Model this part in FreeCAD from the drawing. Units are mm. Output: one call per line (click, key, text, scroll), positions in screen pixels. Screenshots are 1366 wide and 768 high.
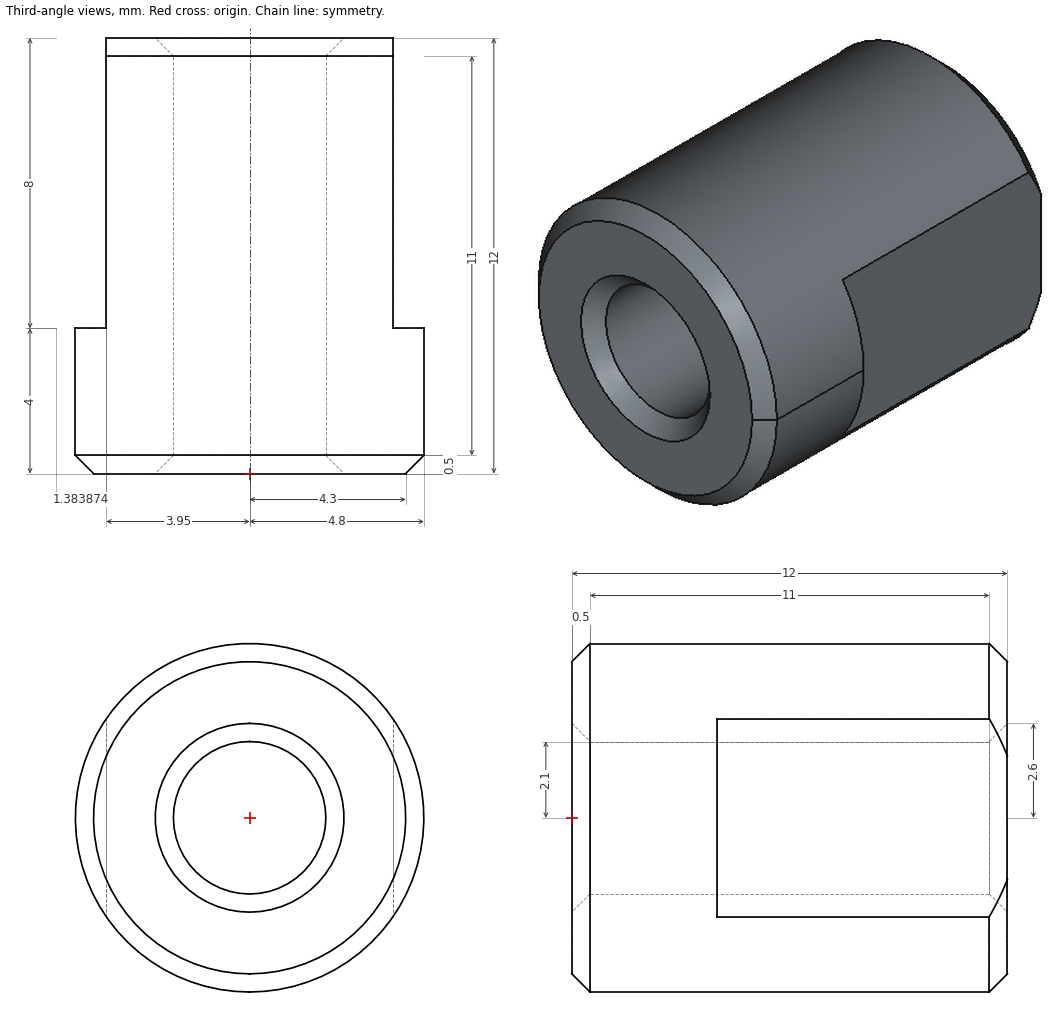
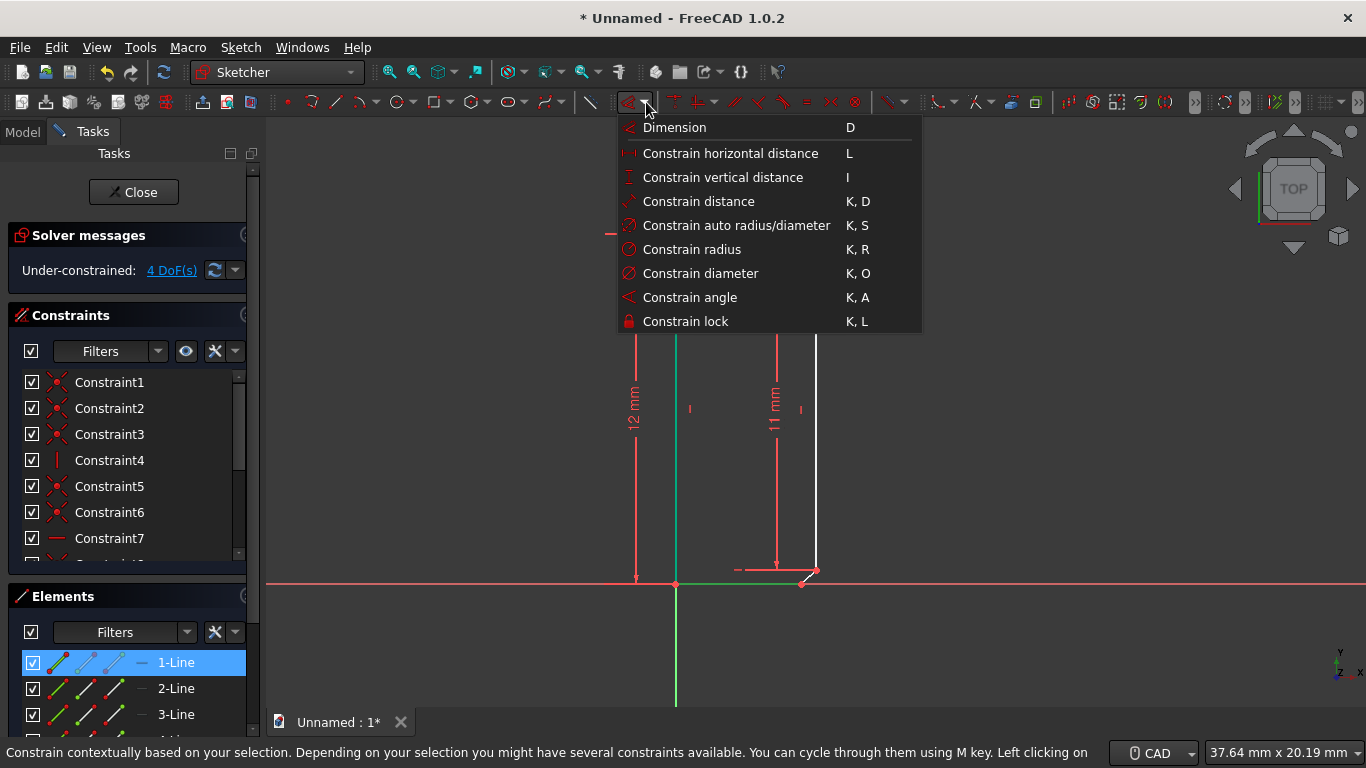
click(770, 153)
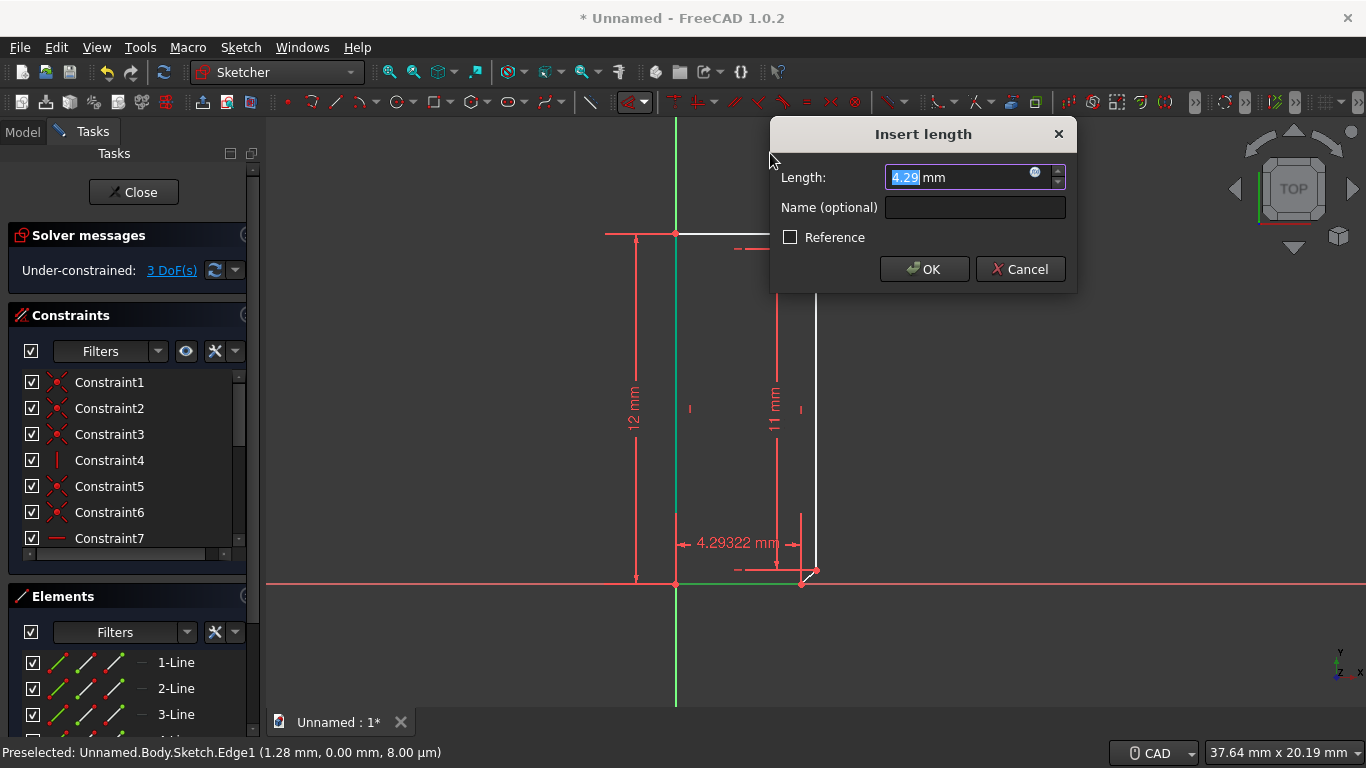
text(4.3)
key(Return)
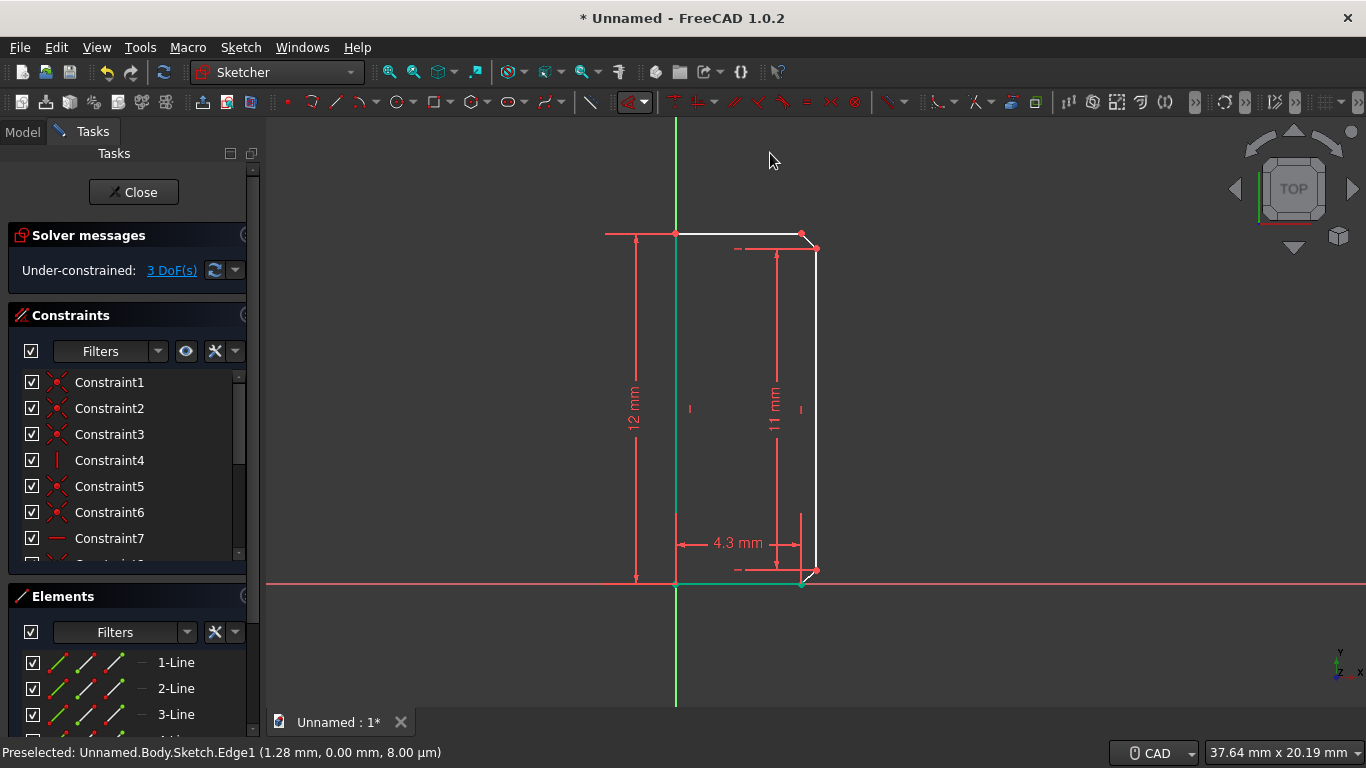
click(763, 234)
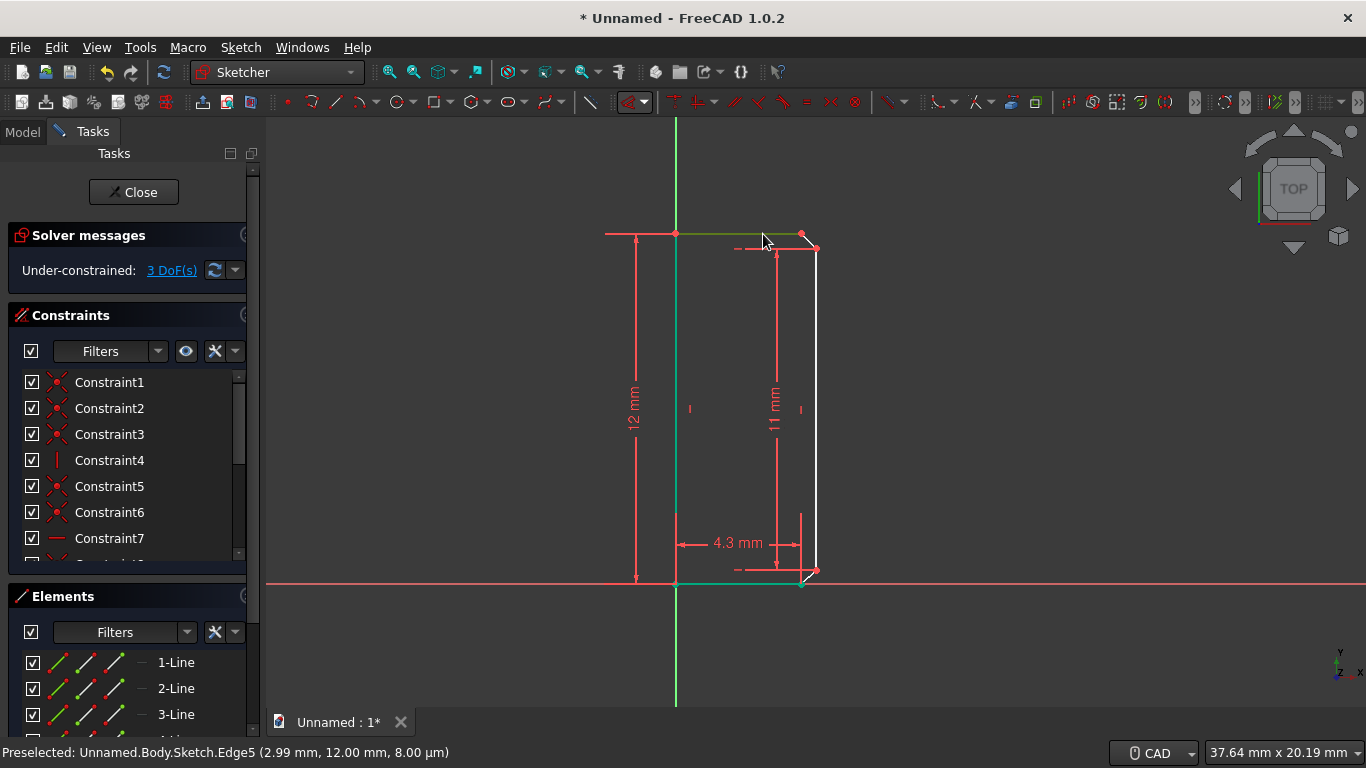
click(646, 102)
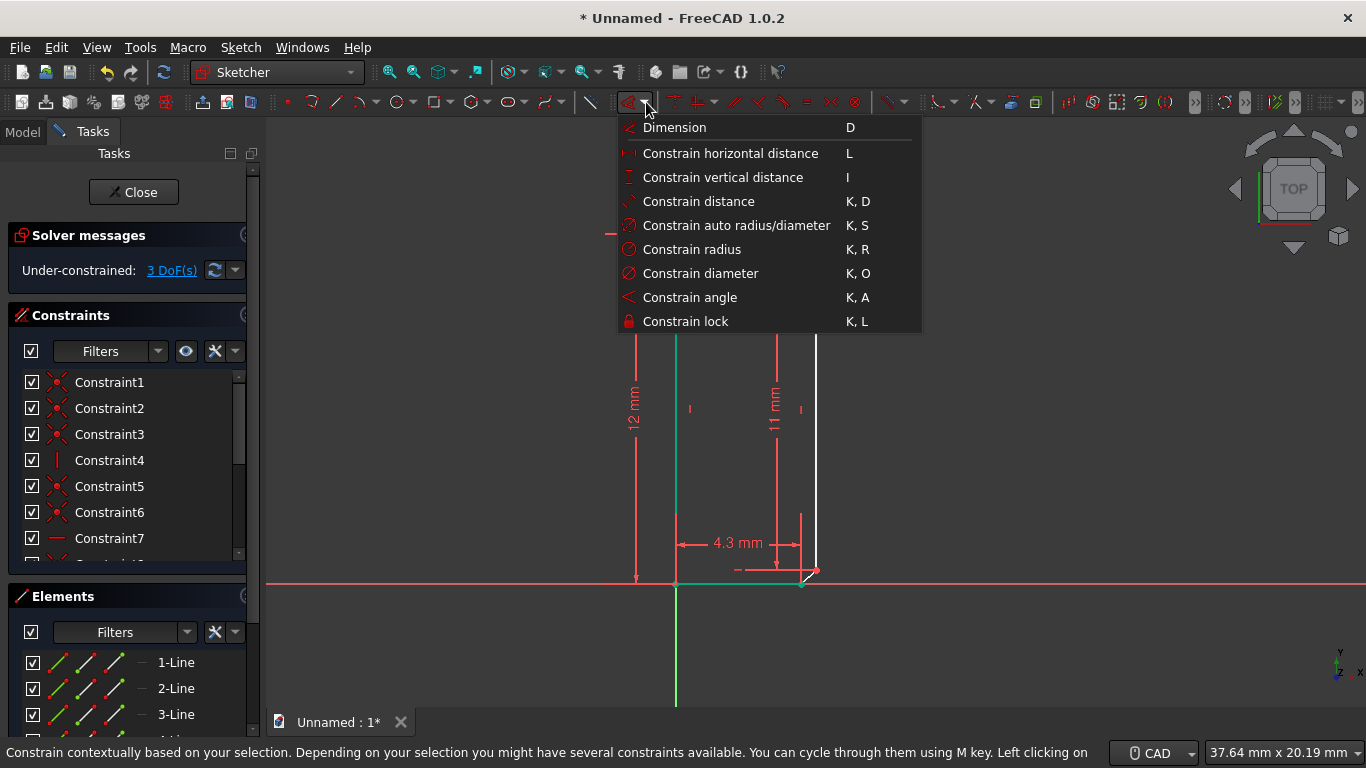
click(770, 153)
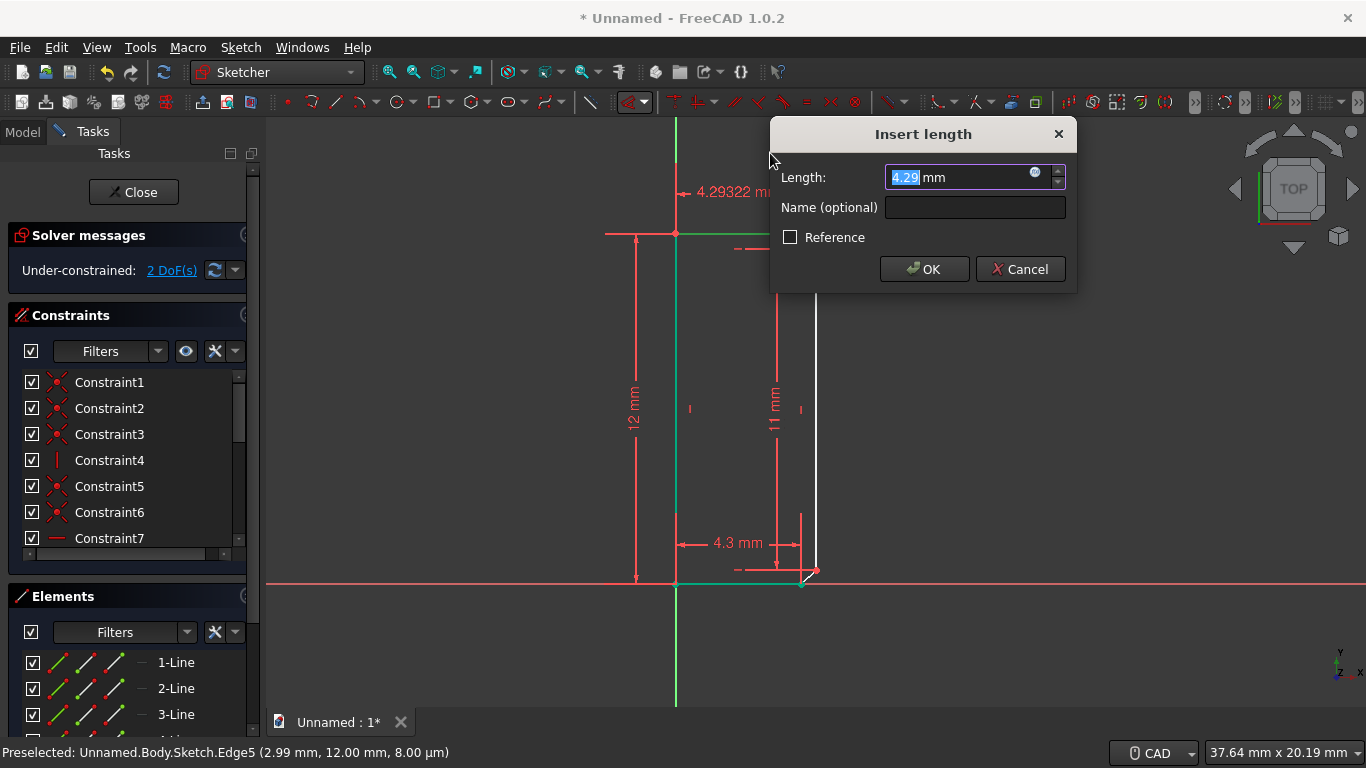
text(4.3)
key(Return)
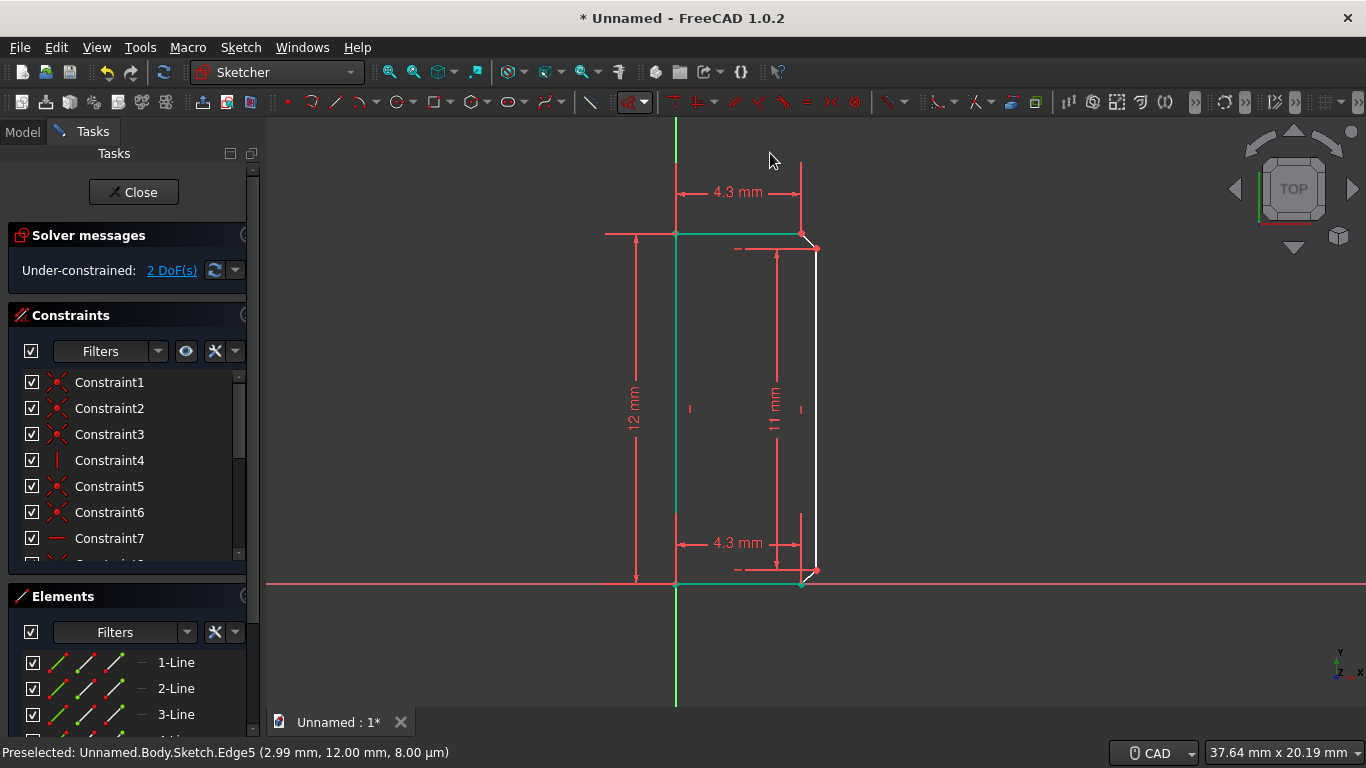
click(816, 570)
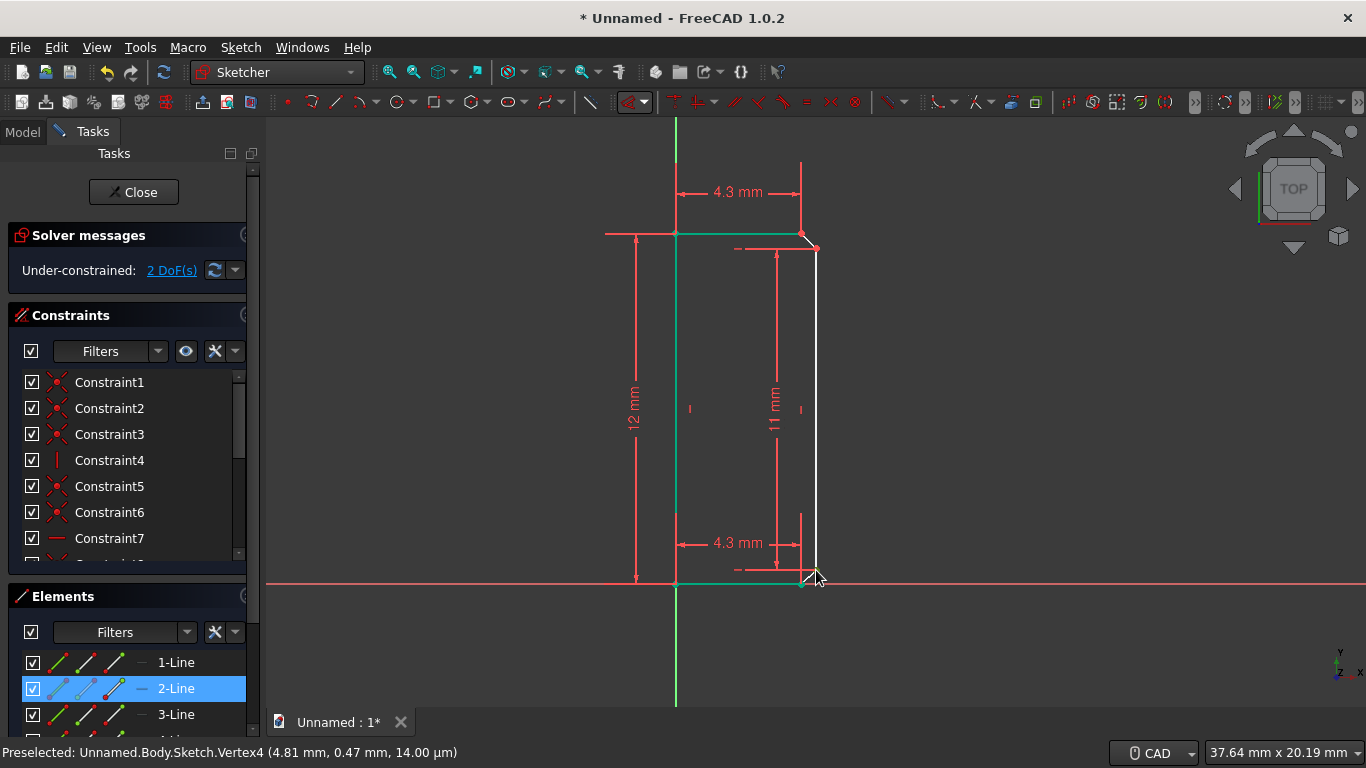
click(646, 102)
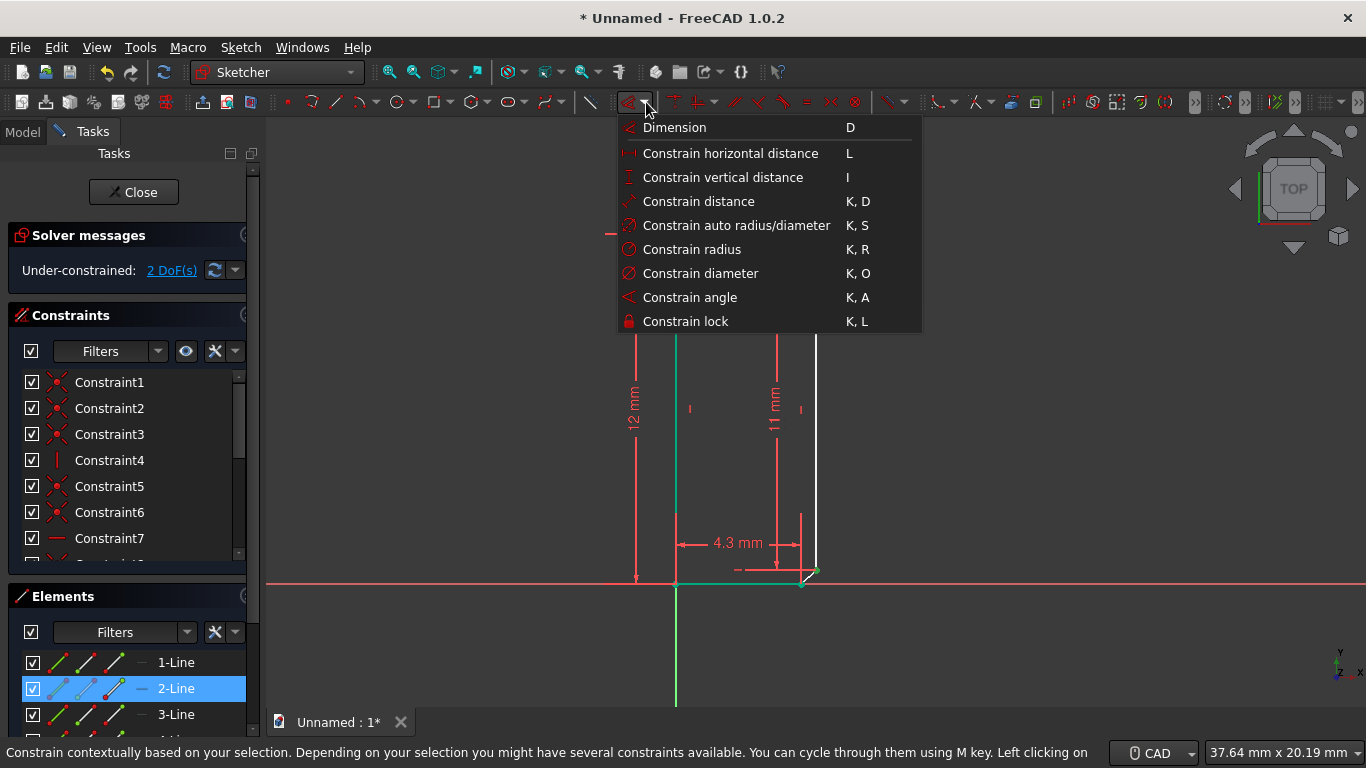
click(770, 153)